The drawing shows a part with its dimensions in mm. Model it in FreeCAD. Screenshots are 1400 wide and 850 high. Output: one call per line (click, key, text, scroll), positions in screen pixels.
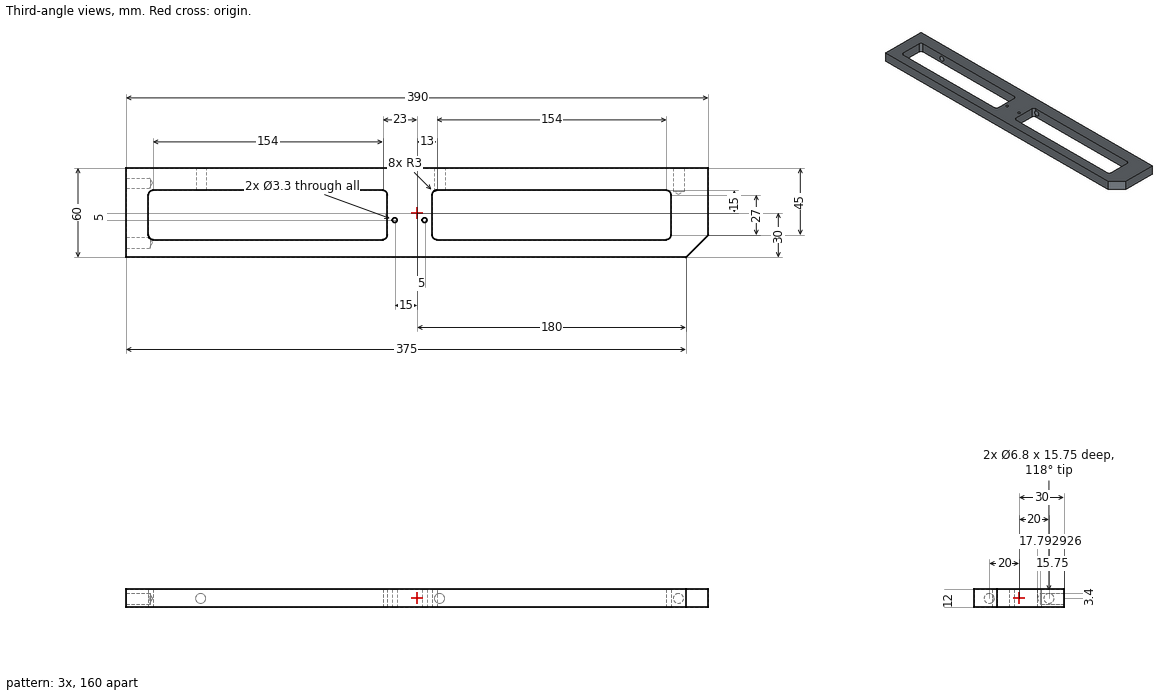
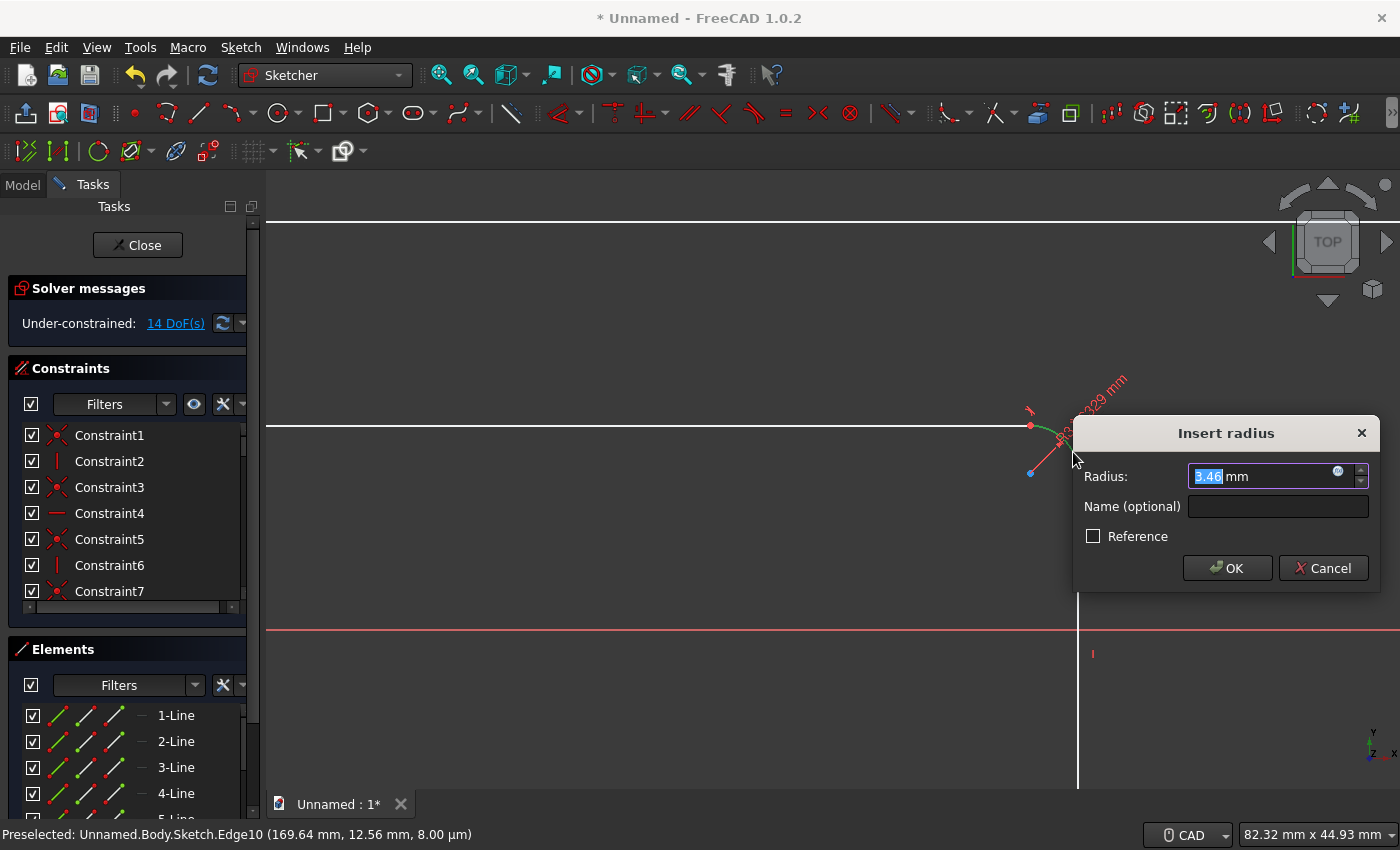
text(3)
key(Return)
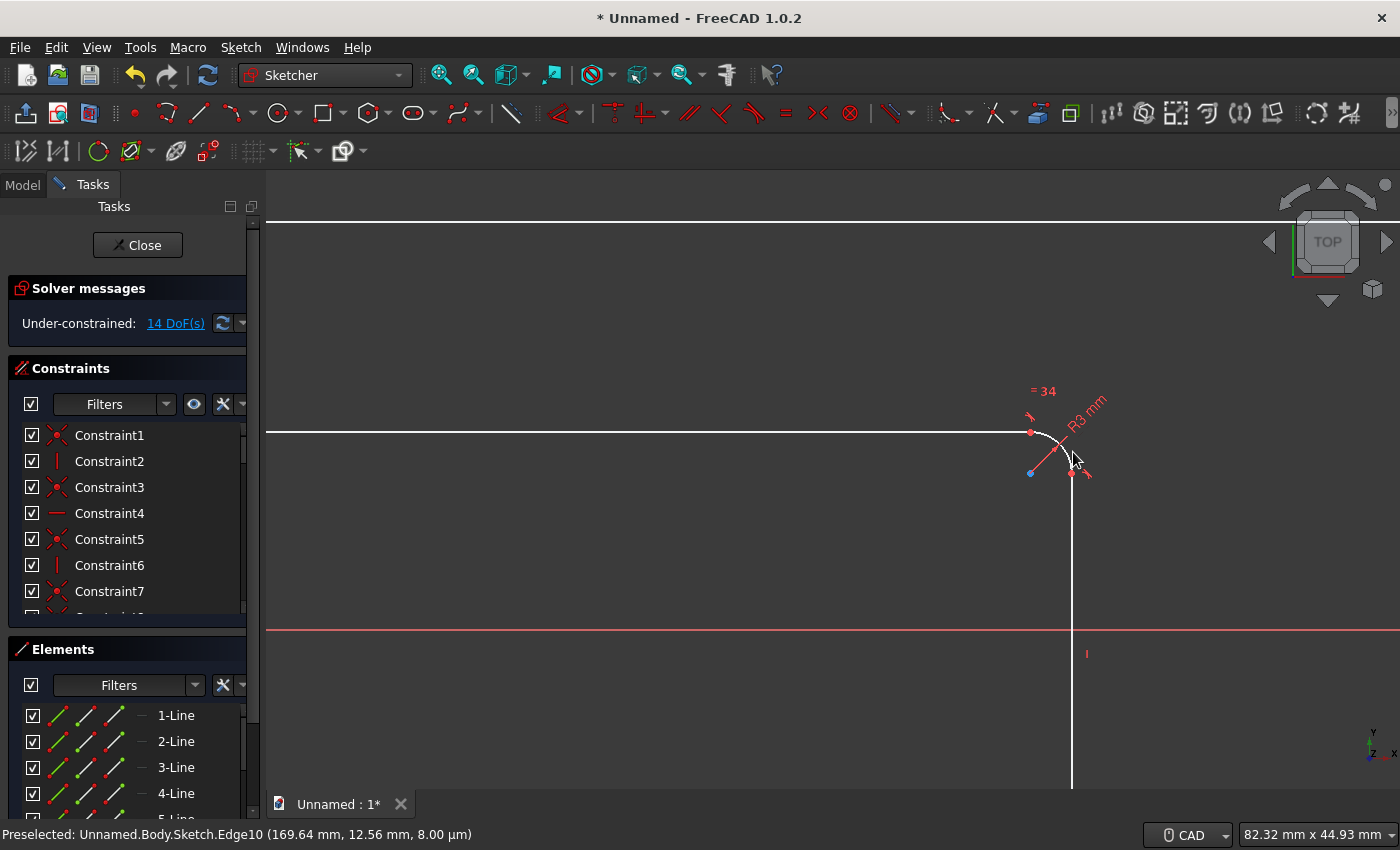
scroll(1082, 456, down, 10)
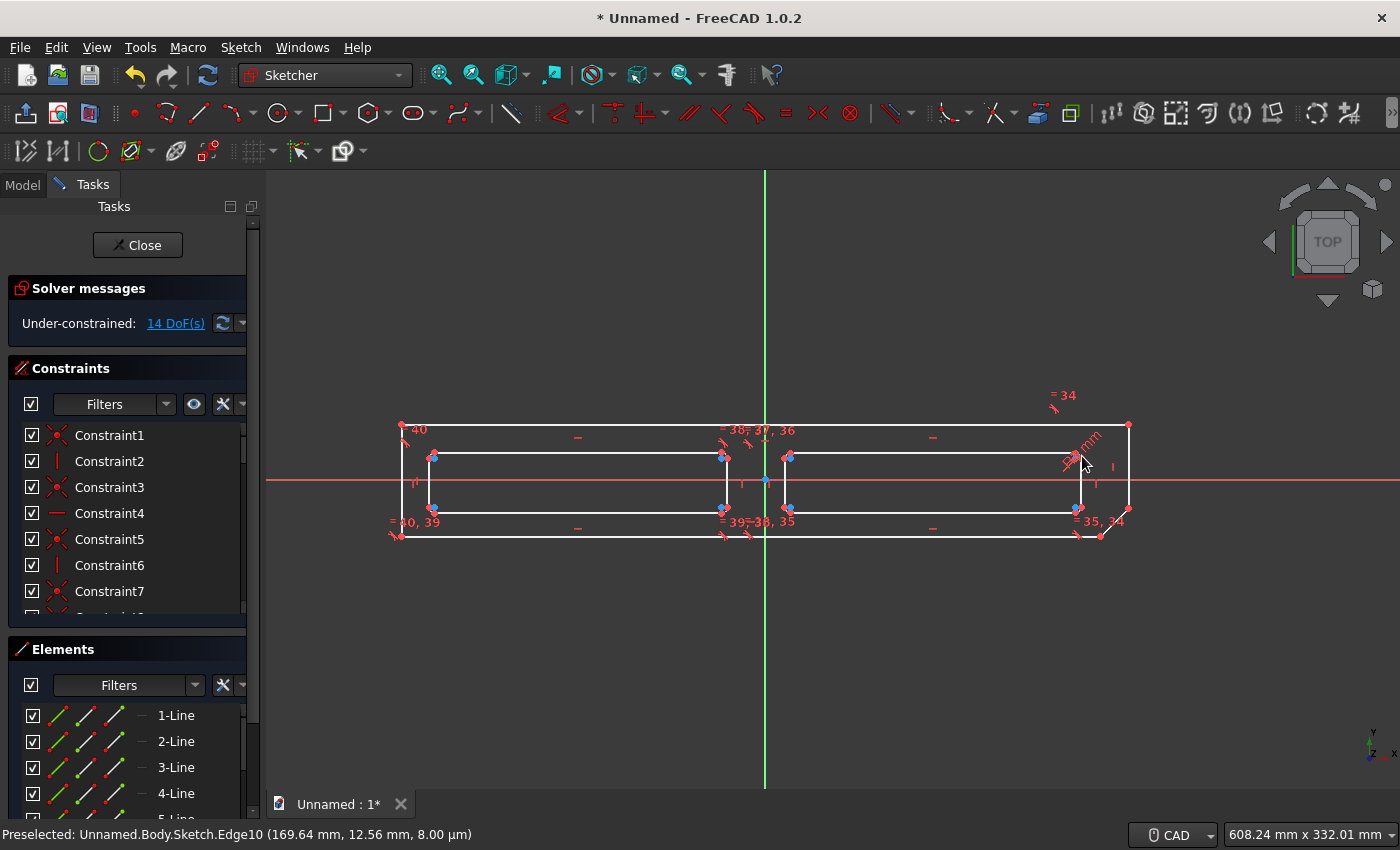
scroll(1129, 484, up, 7)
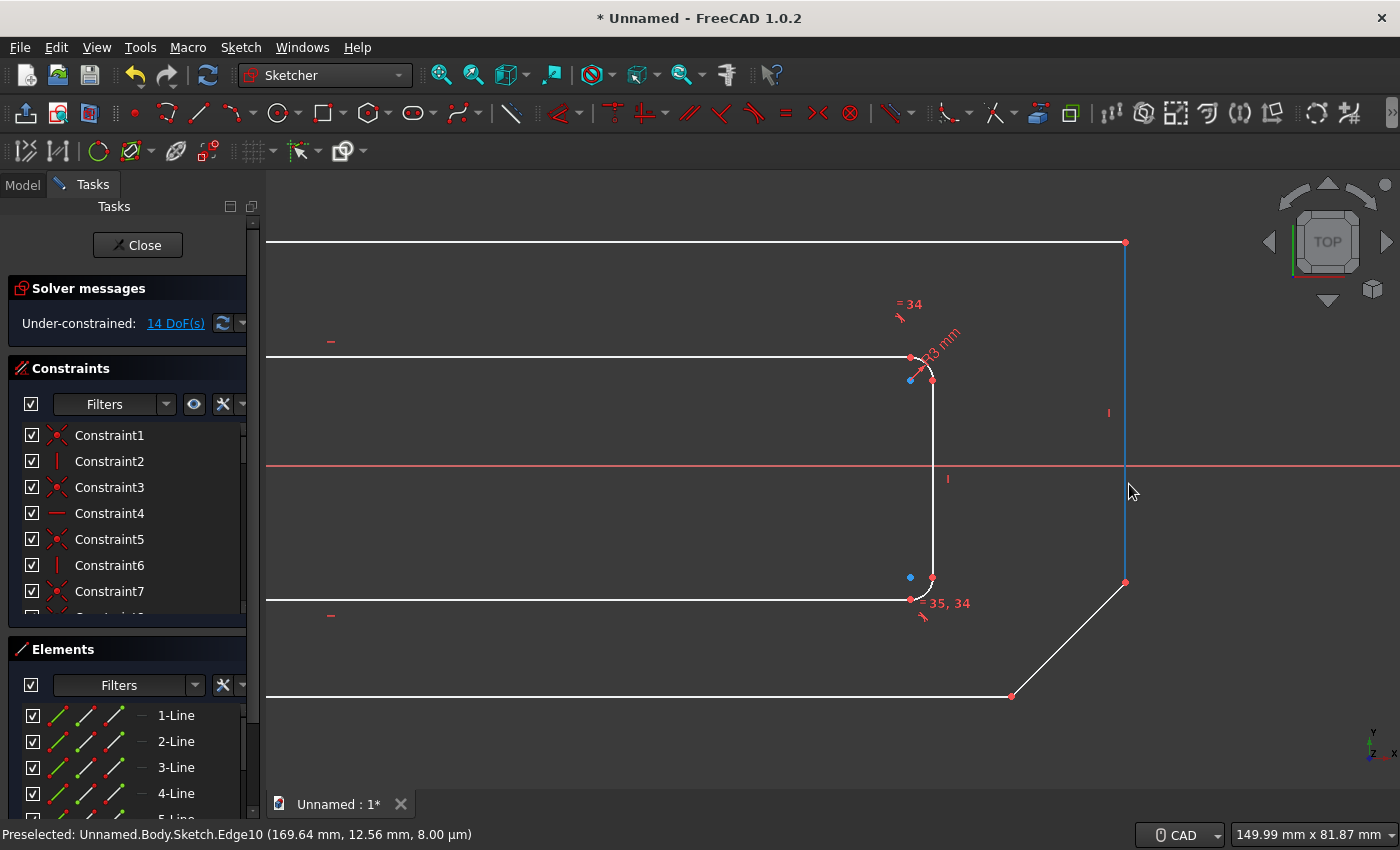
click(1125, 481)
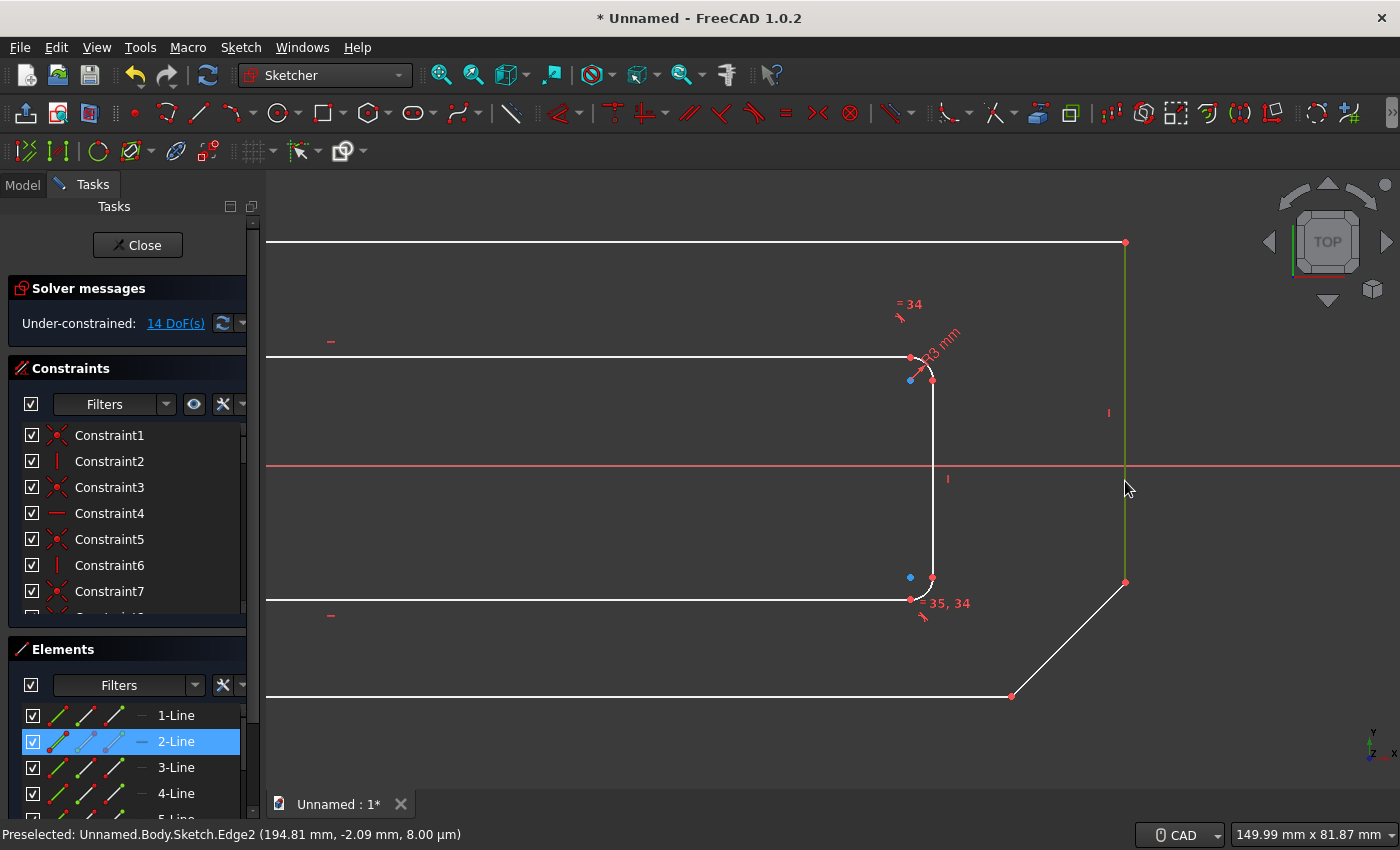
click(582, 114)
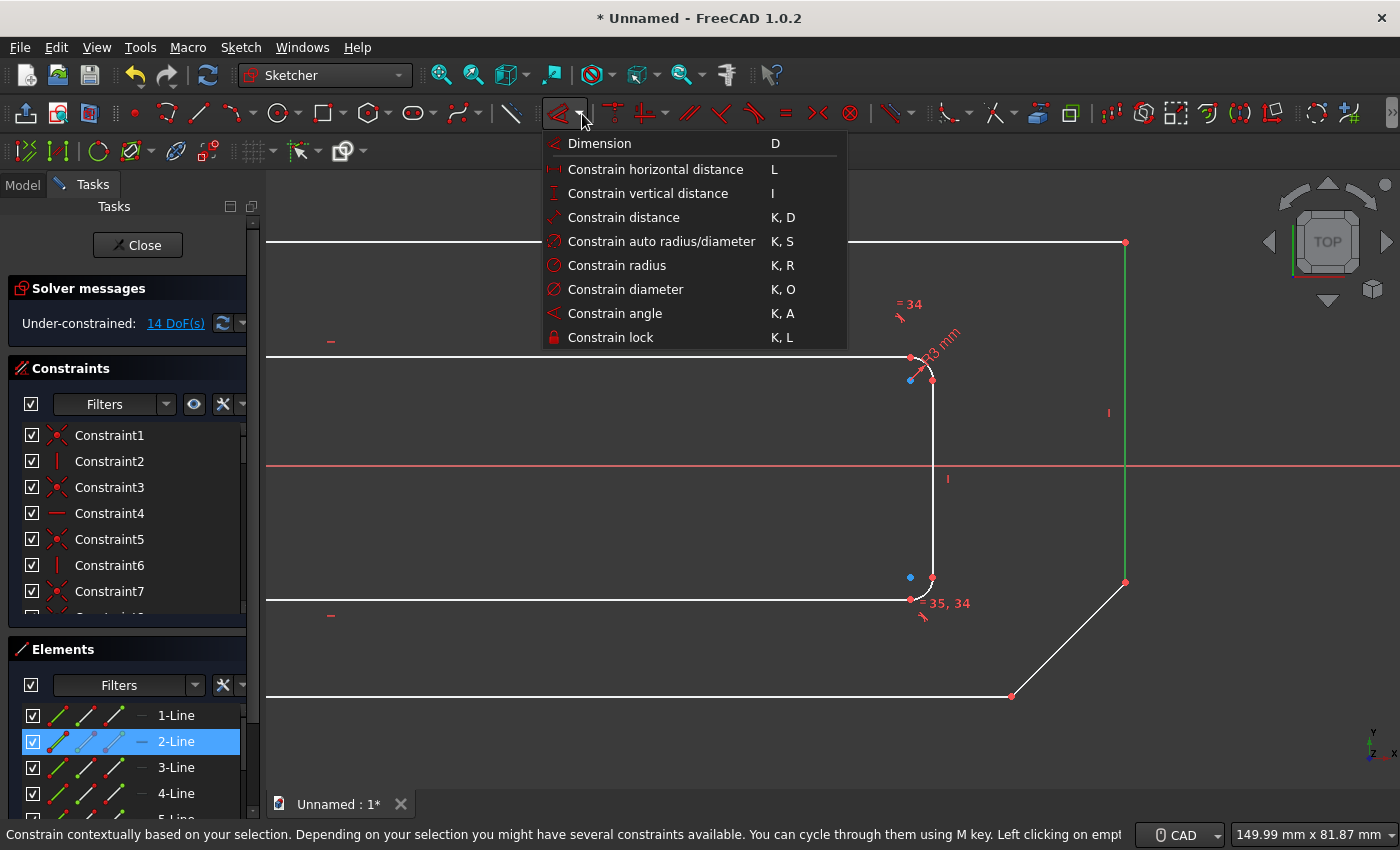
click(695, 193)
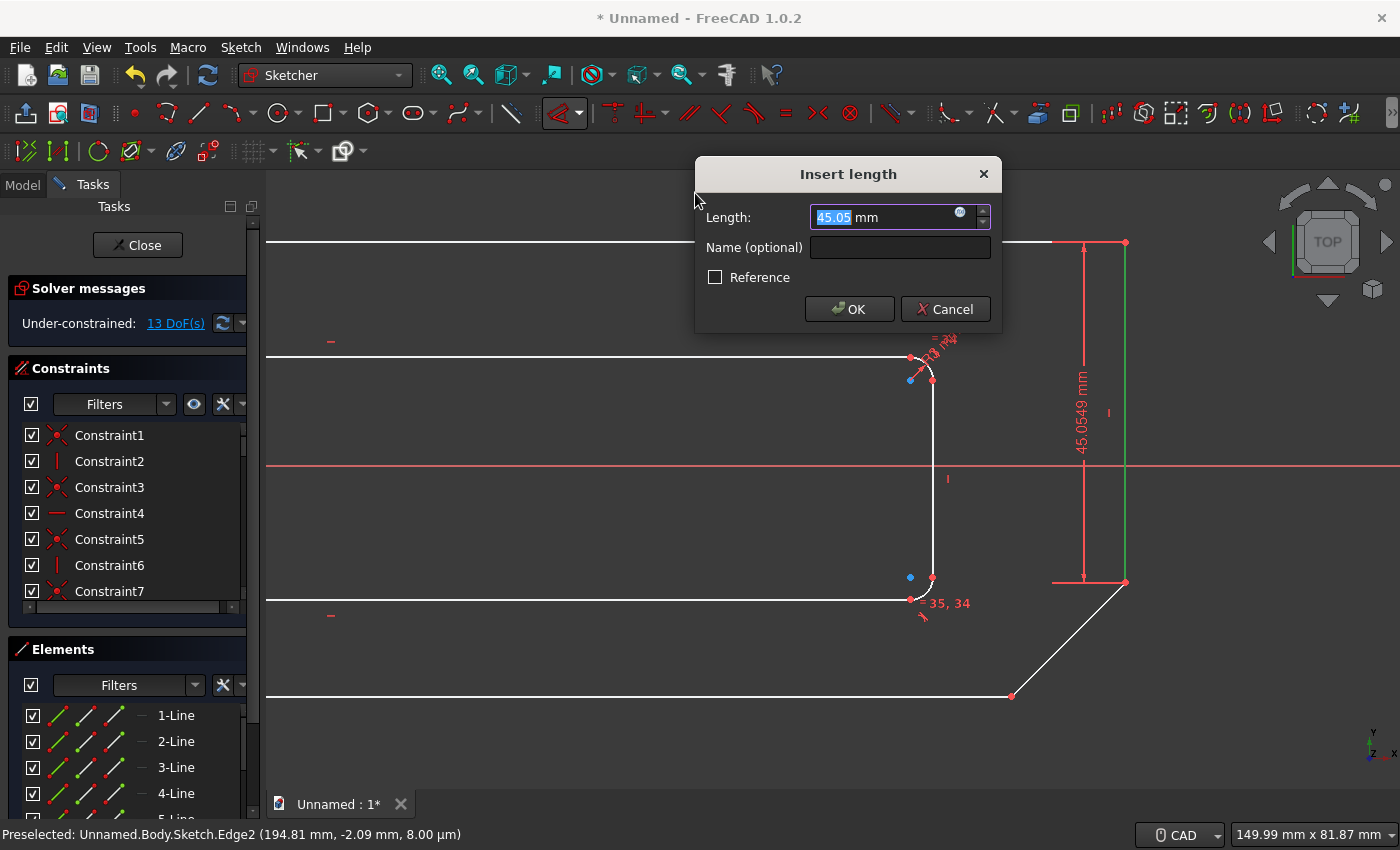
text(45)
key(Return)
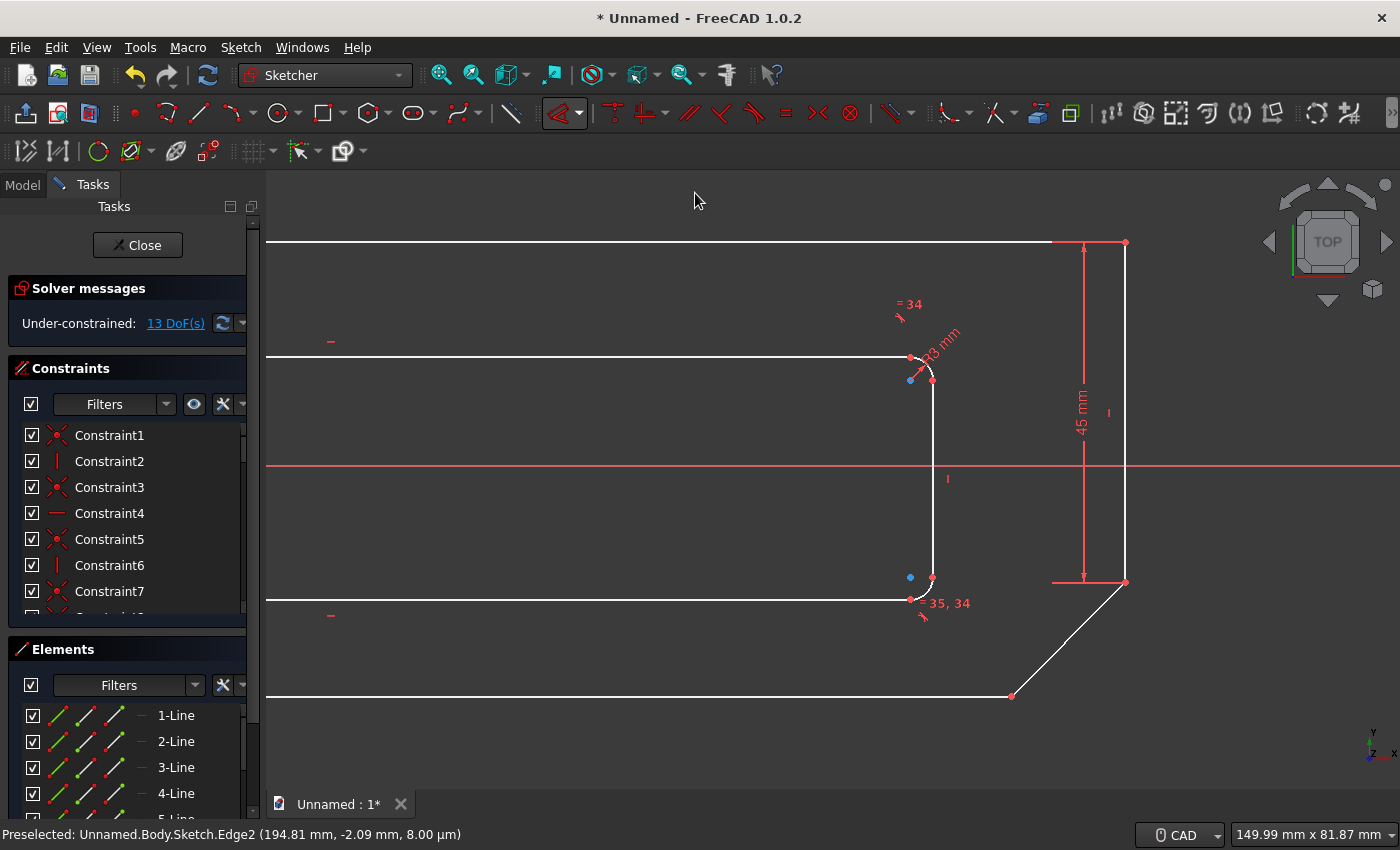
scroll(1129, 484, down, 7)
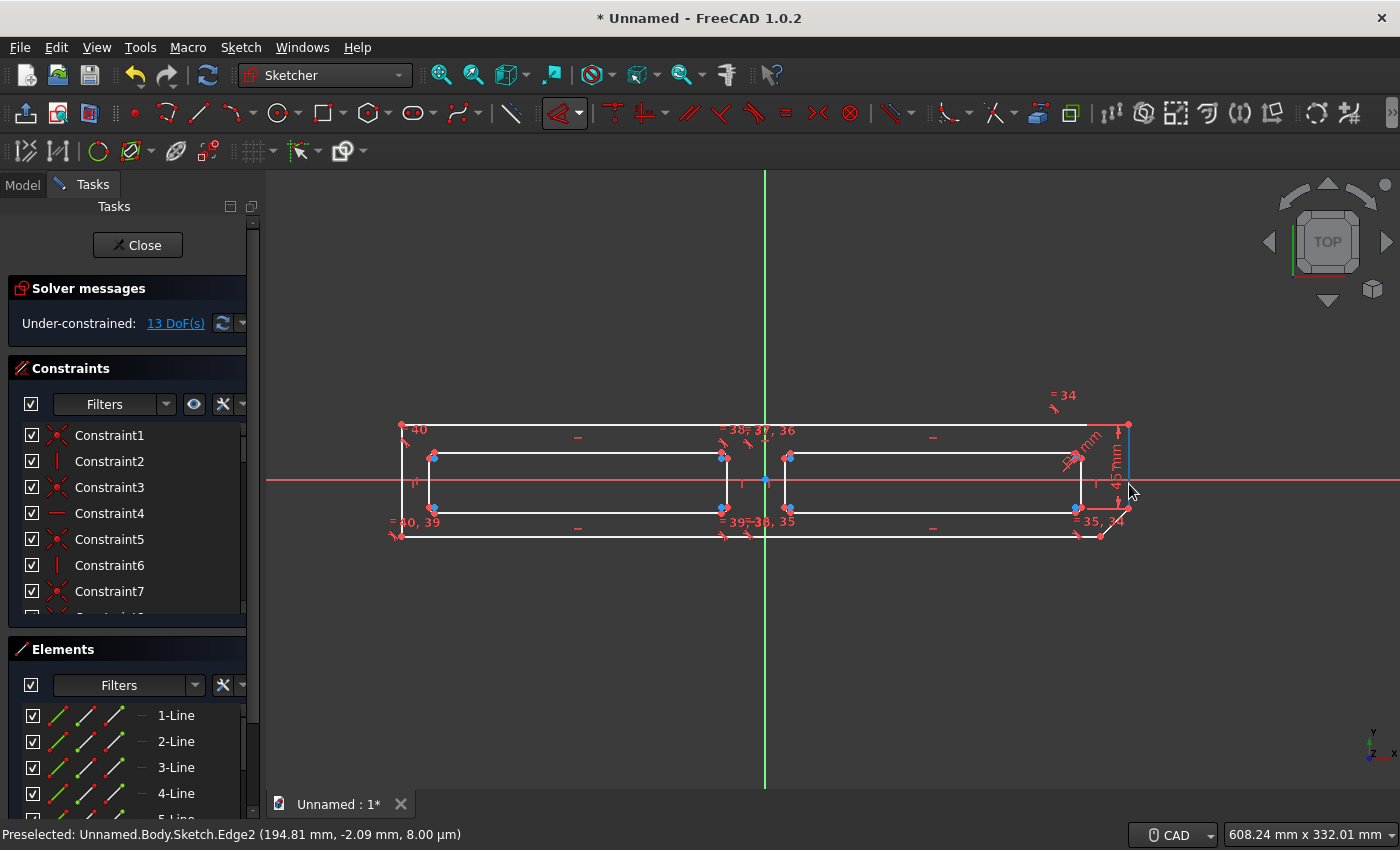
click(402, 458)